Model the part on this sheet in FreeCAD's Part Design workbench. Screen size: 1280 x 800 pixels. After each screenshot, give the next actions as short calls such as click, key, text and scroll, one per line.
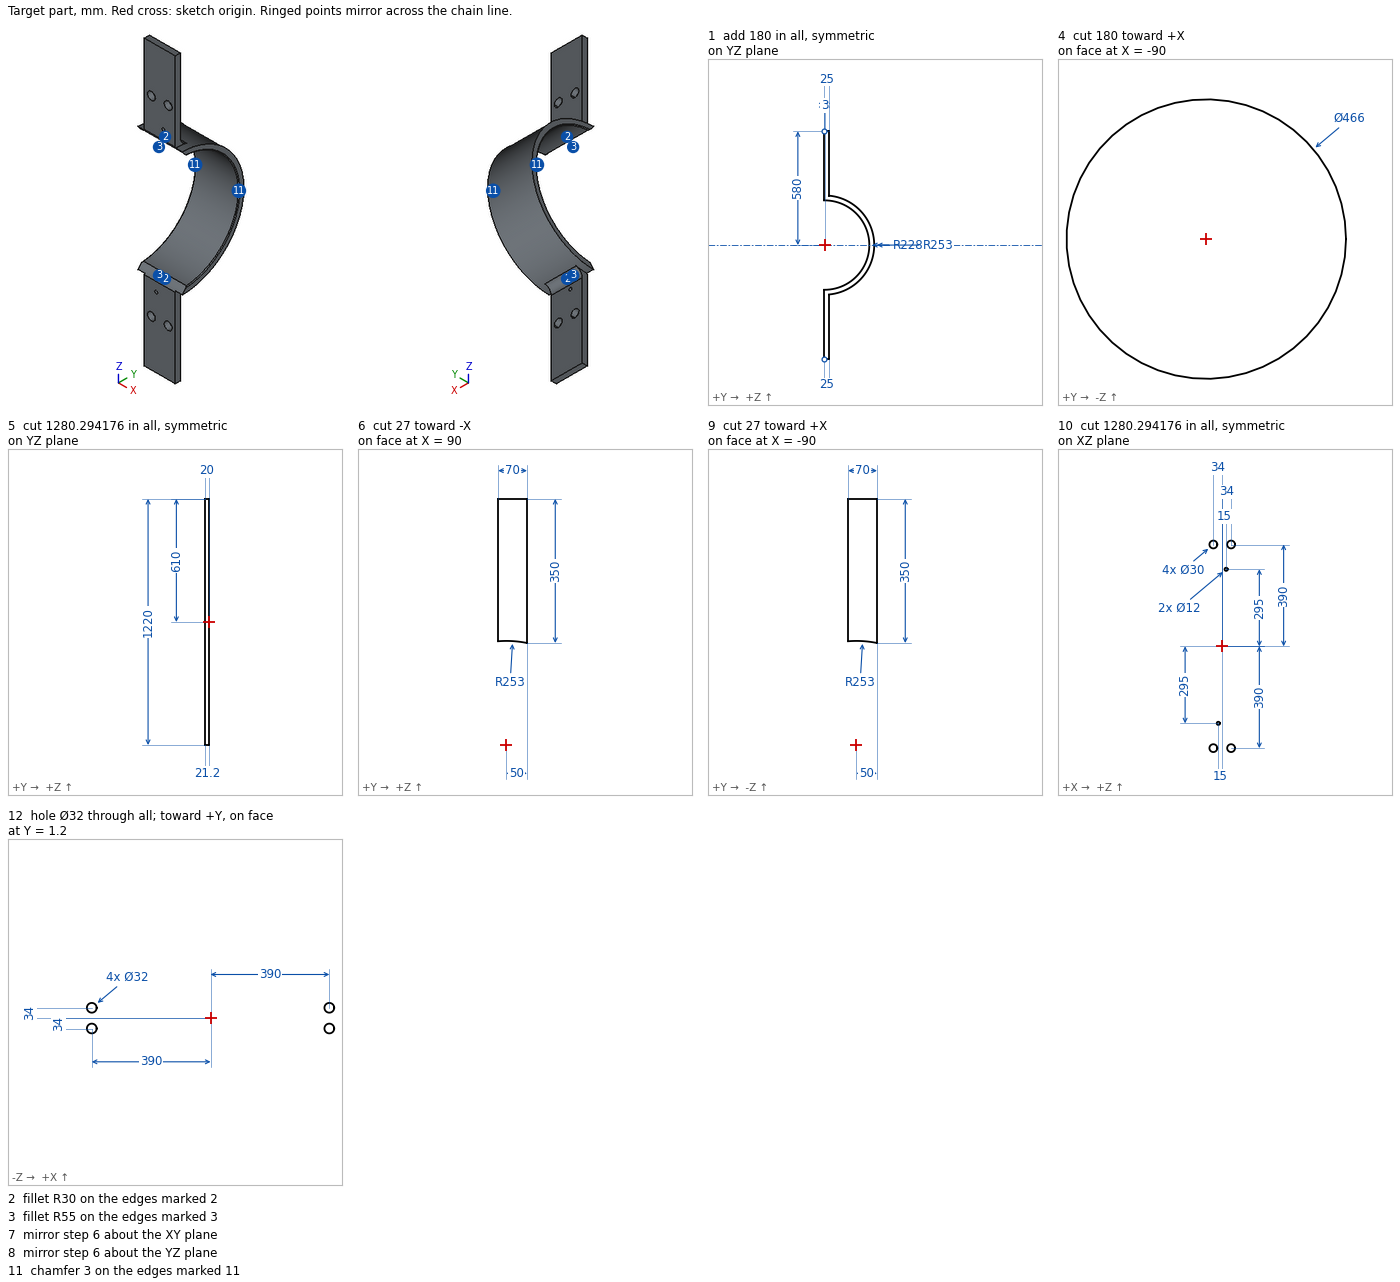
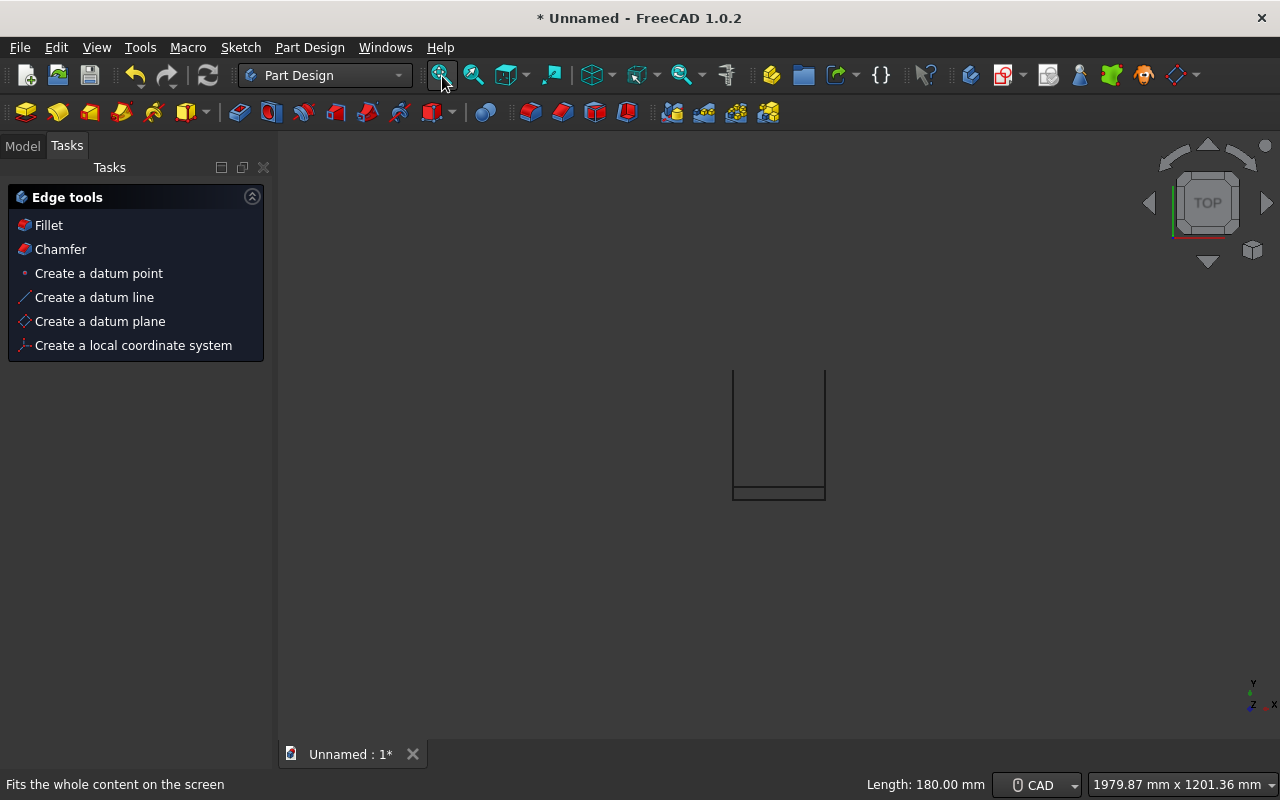
scroll(779, 486, up, 6)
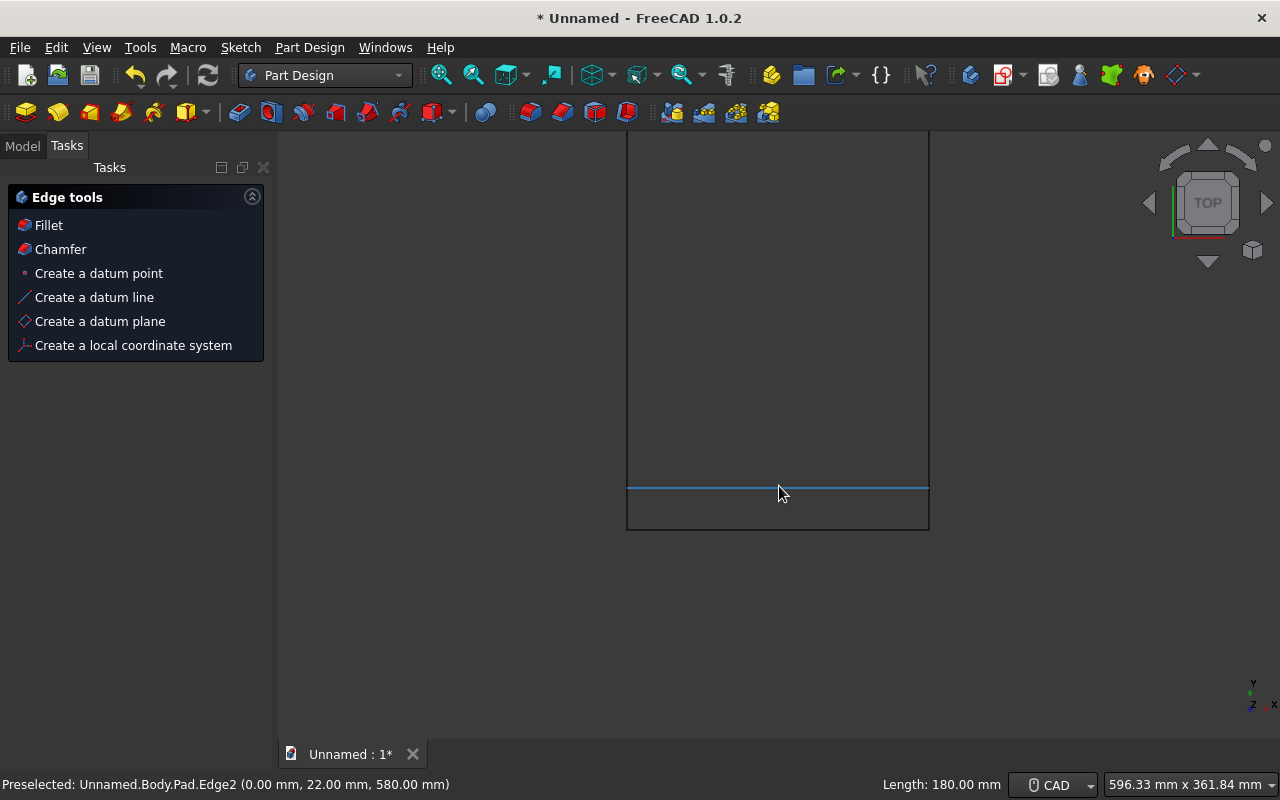
click(442, 76)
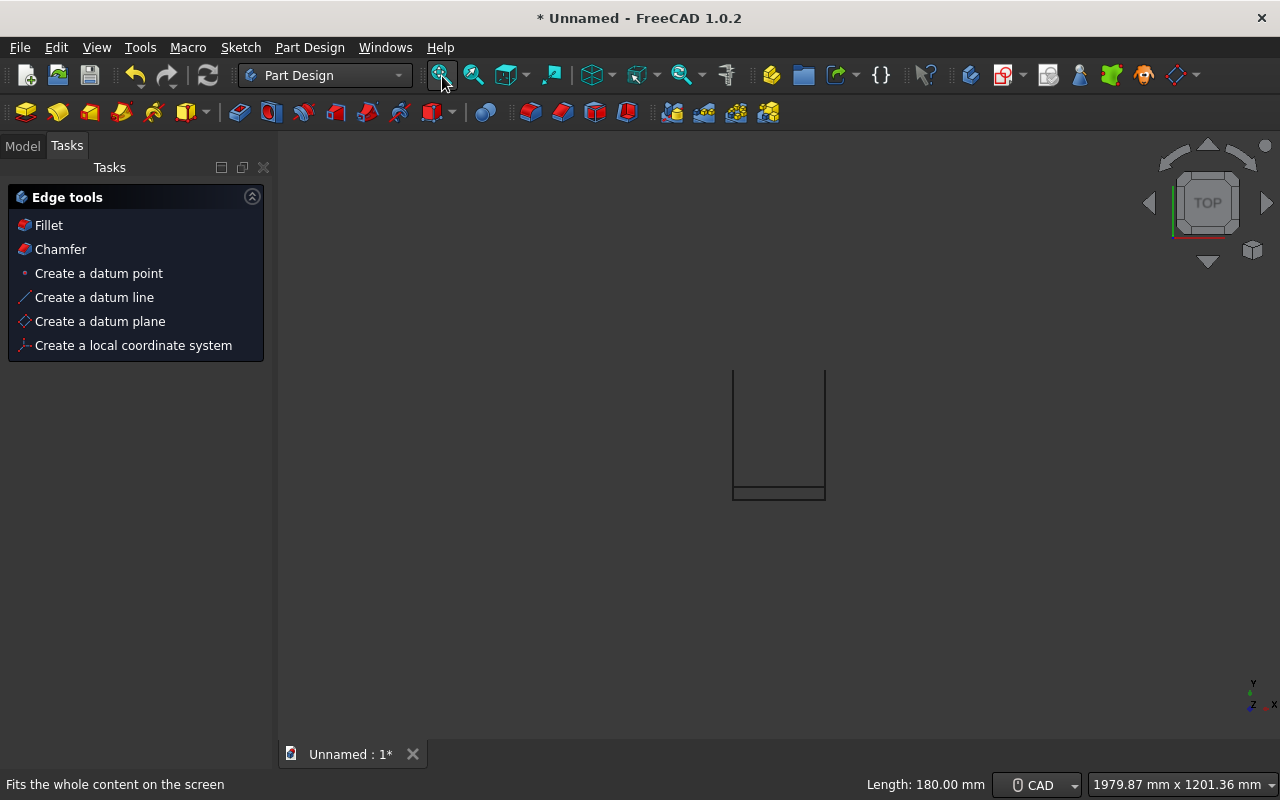
key(1)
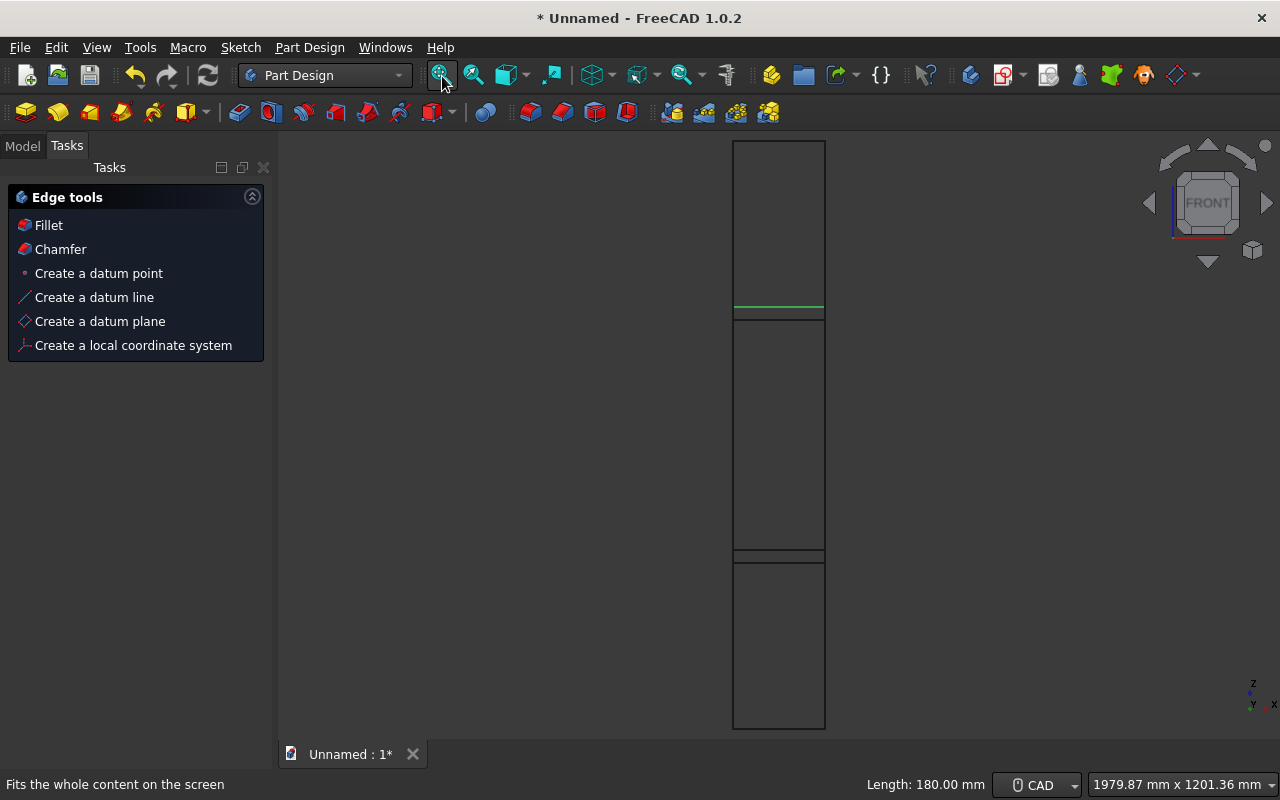
click(779, 562, ctrl)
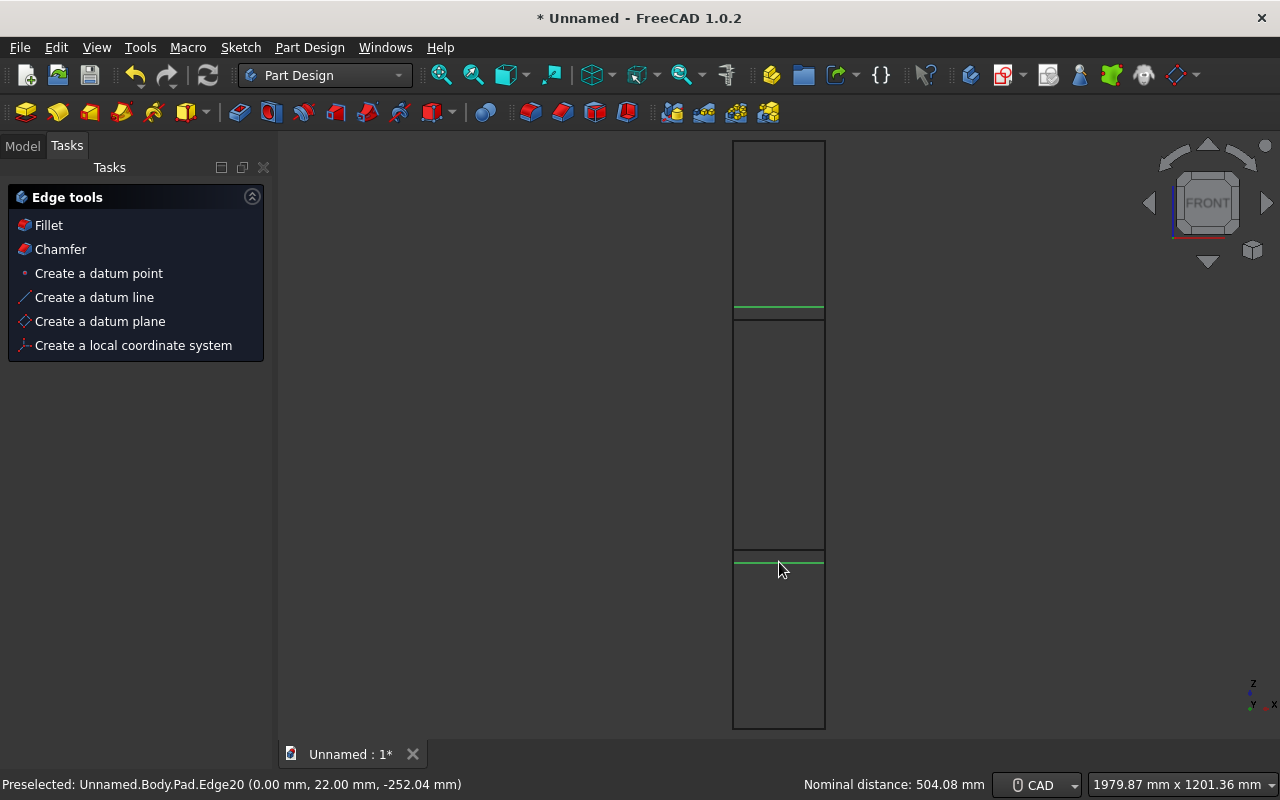
key(v)
key(1)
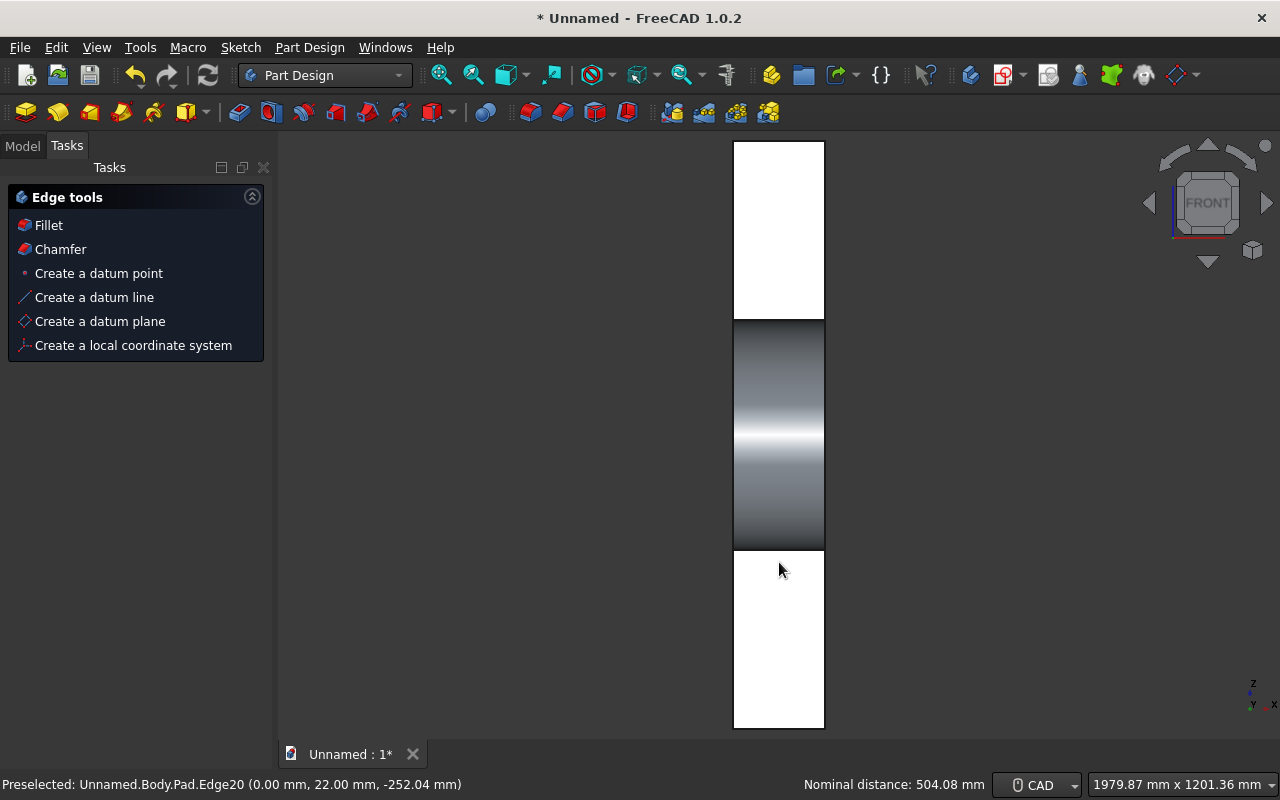
click(532, 112)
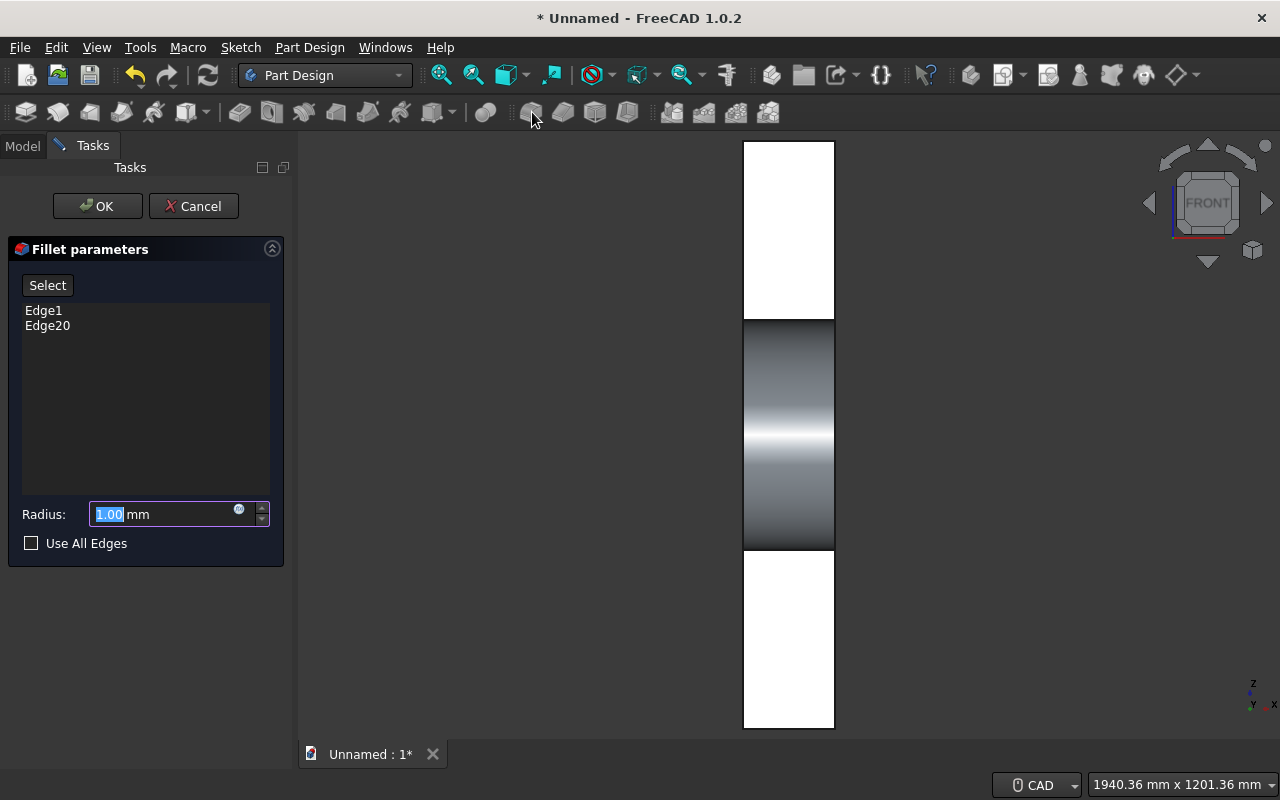
text(30)
key(Tab)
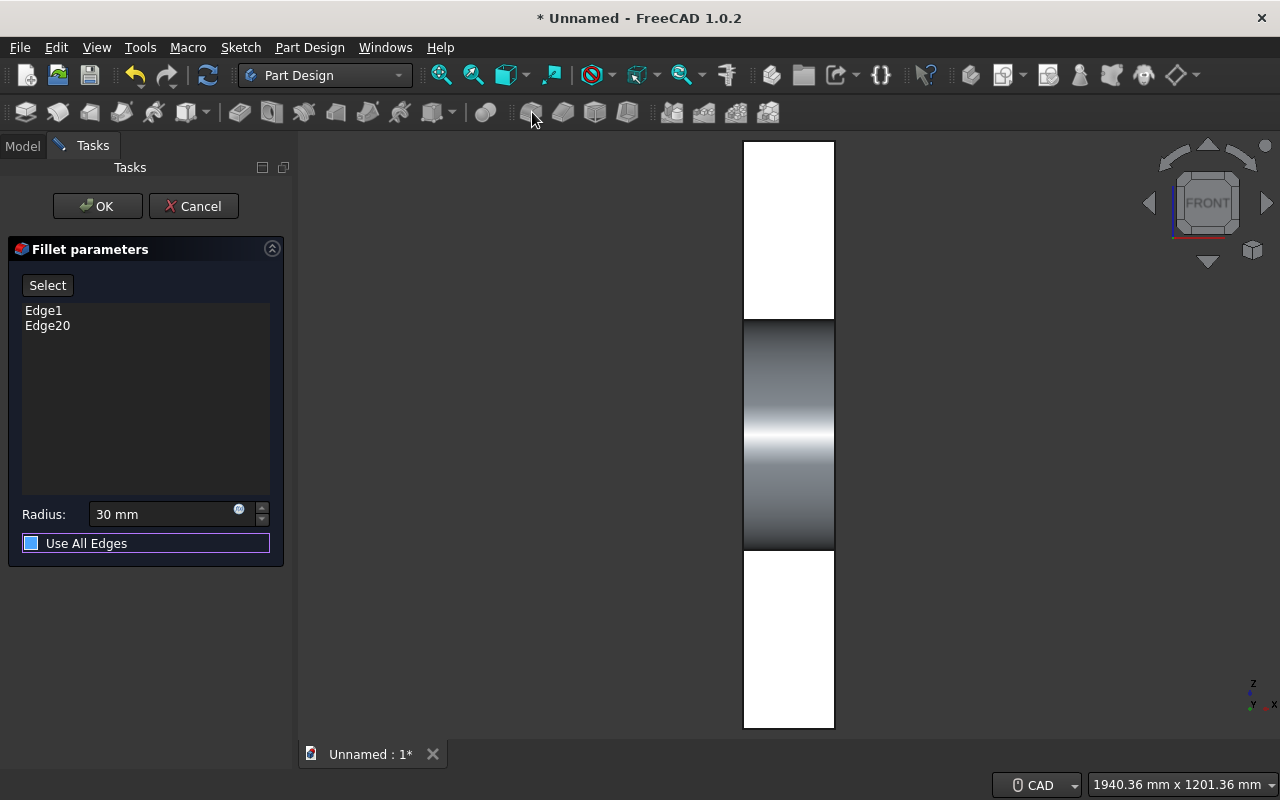
click(98, 206)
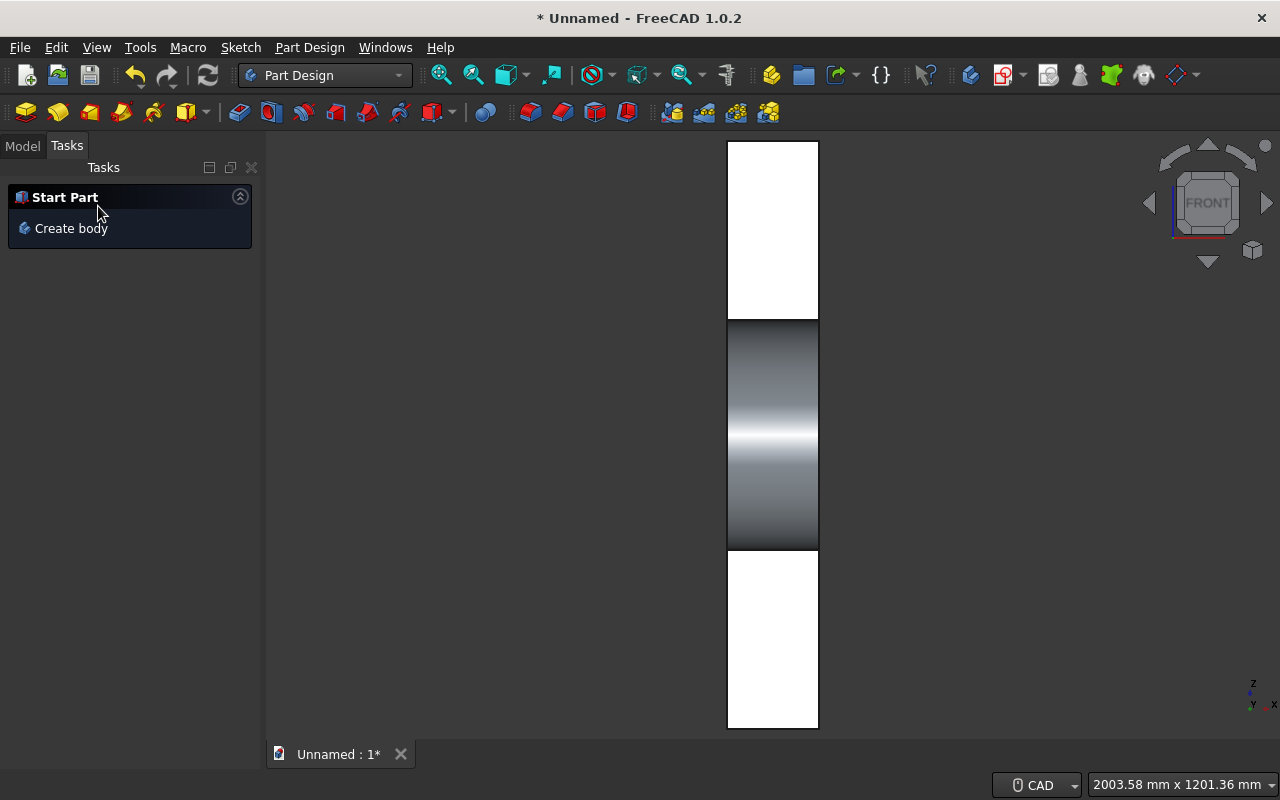
click(773, 549)